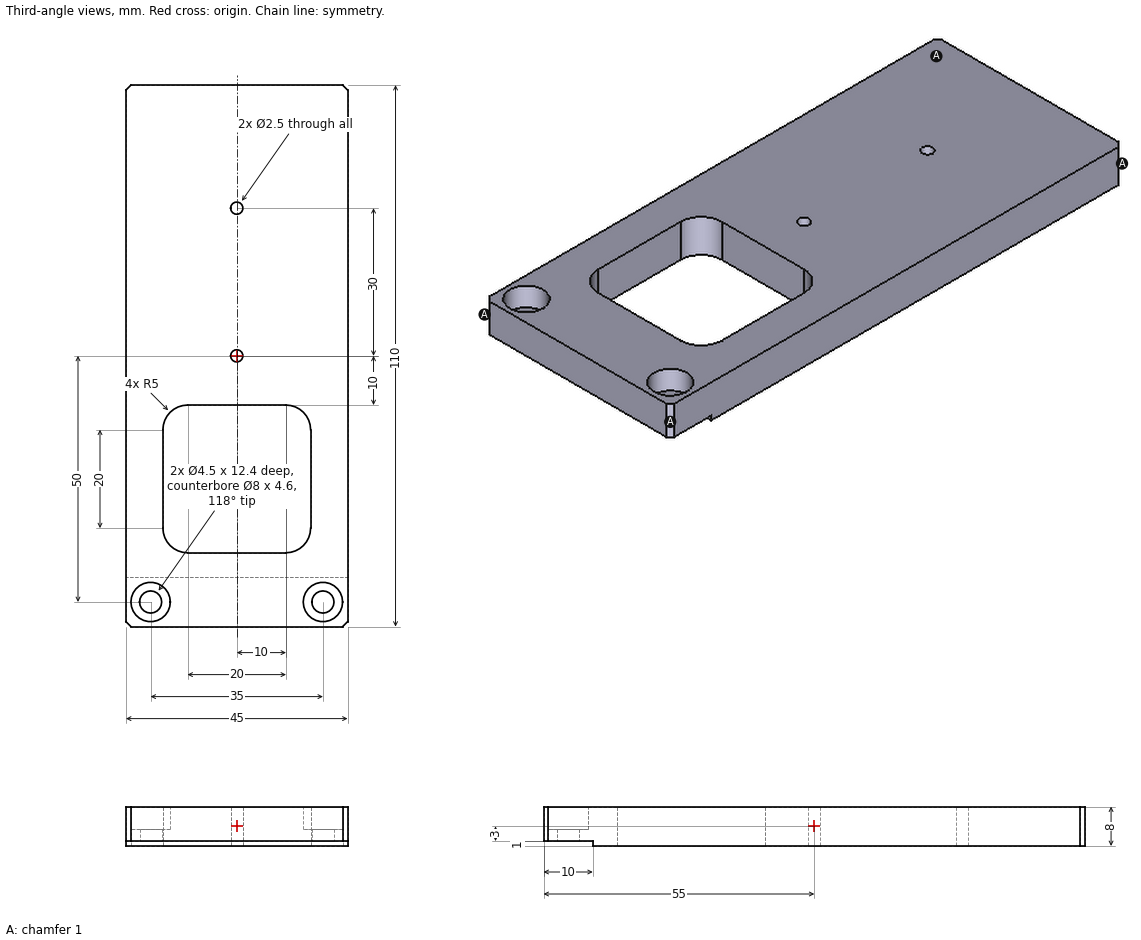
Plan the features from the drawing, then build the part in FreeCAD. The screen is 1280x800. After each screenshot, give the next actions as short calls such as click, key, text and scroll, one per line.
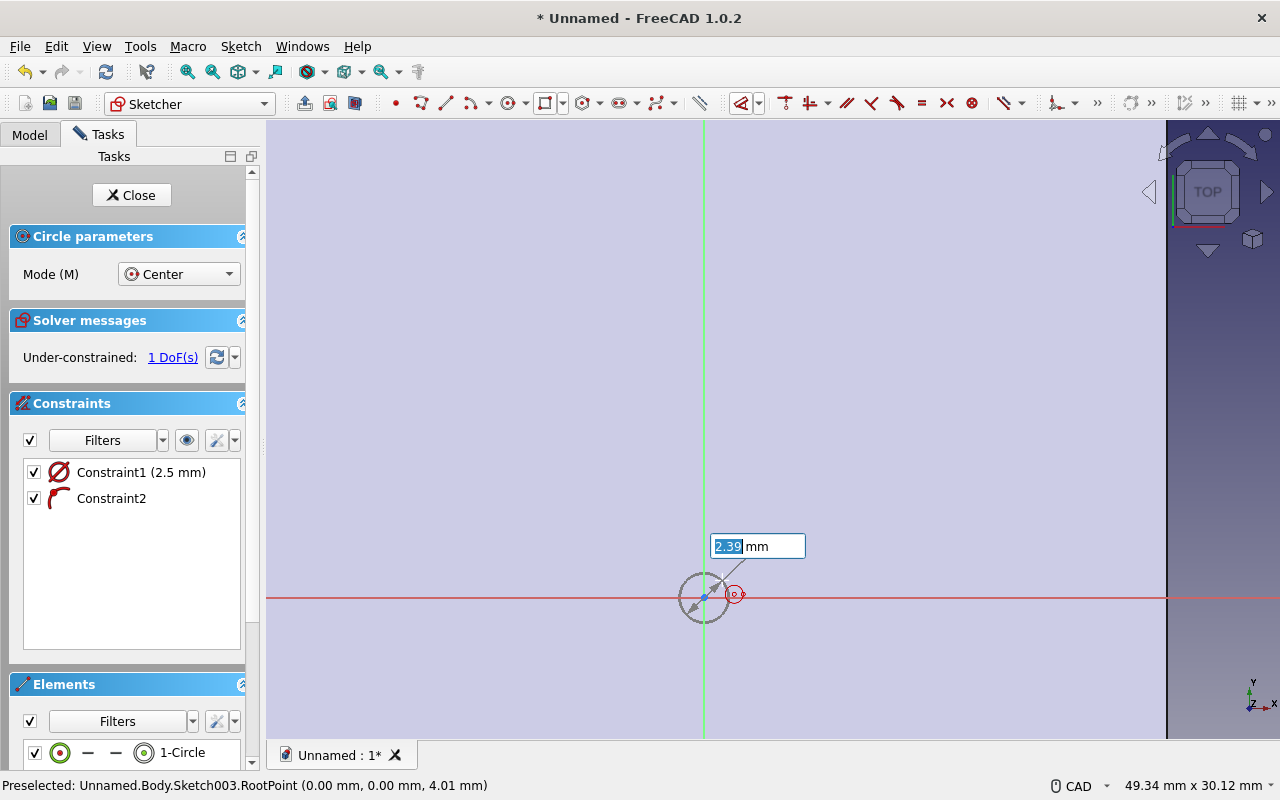
text(2.5)
key(Return)
key(Escape)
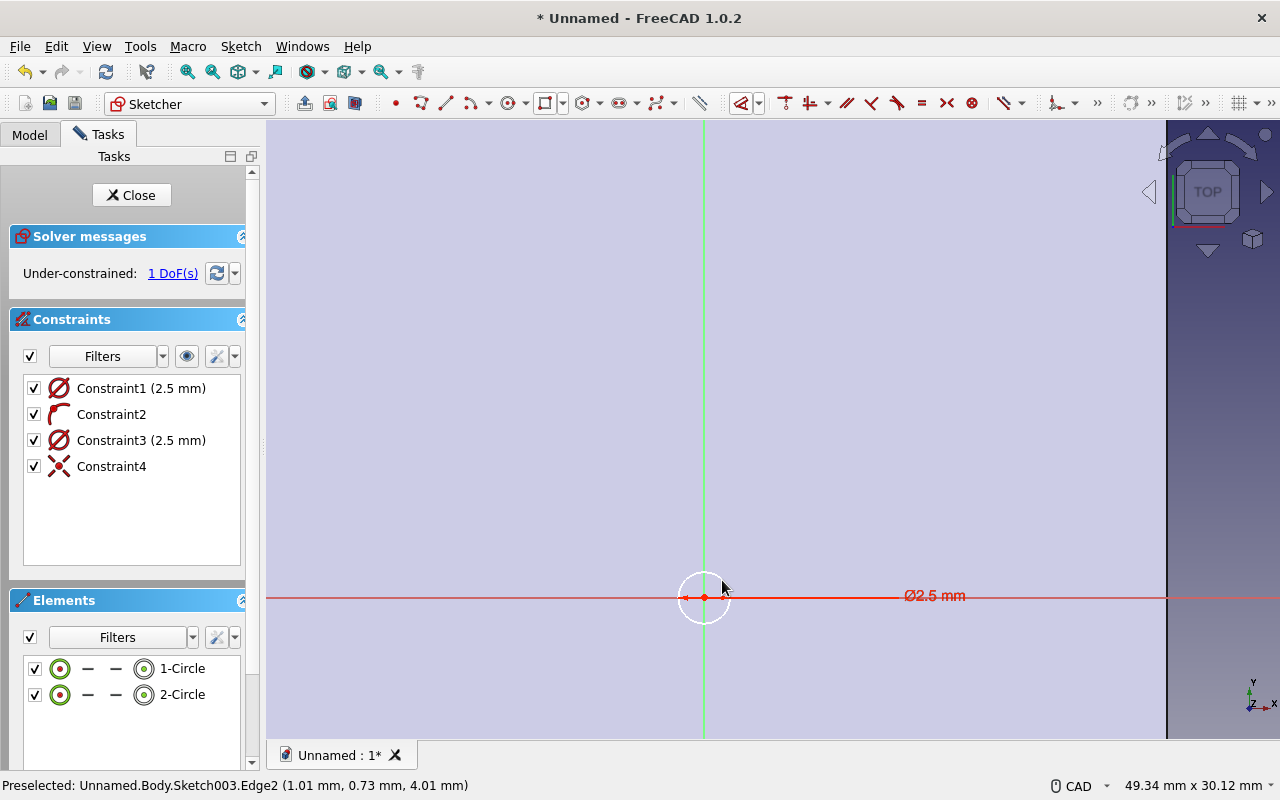
scroll(705, 600, down, 3)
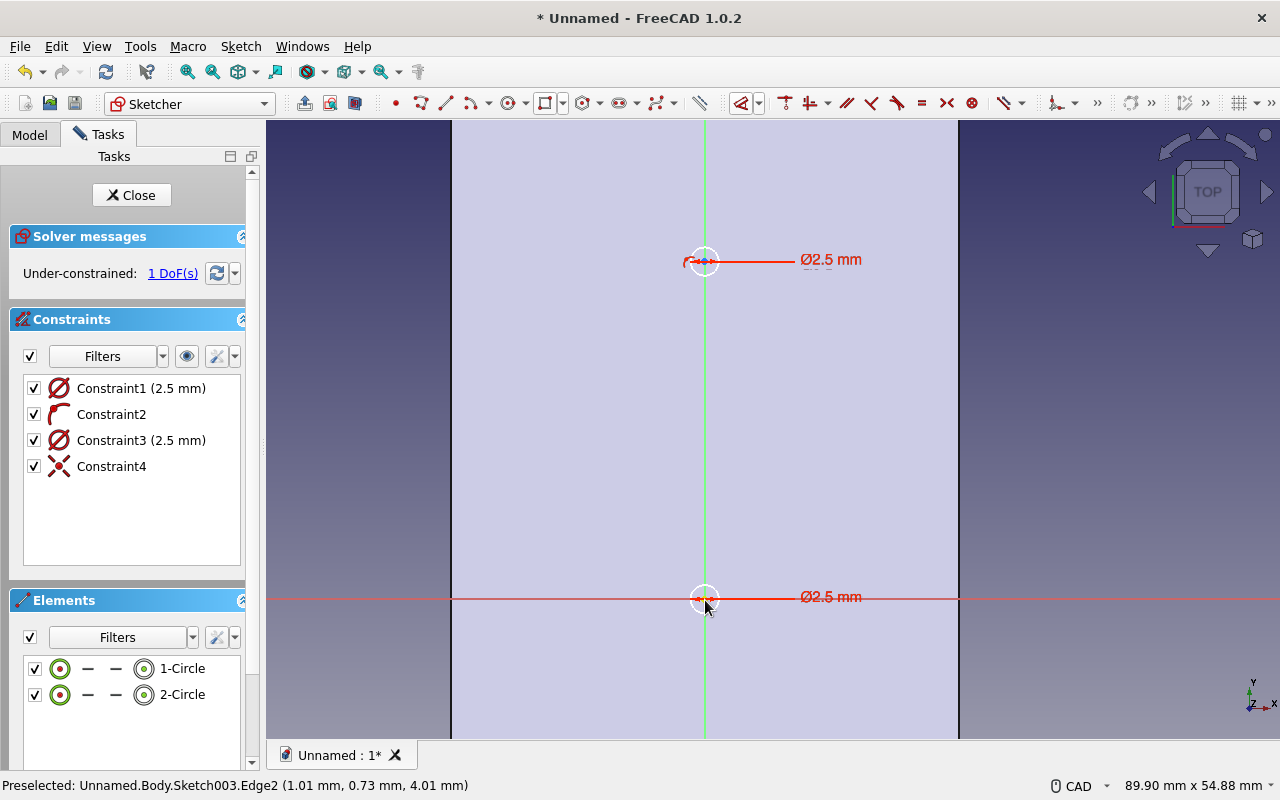
click(705, 262)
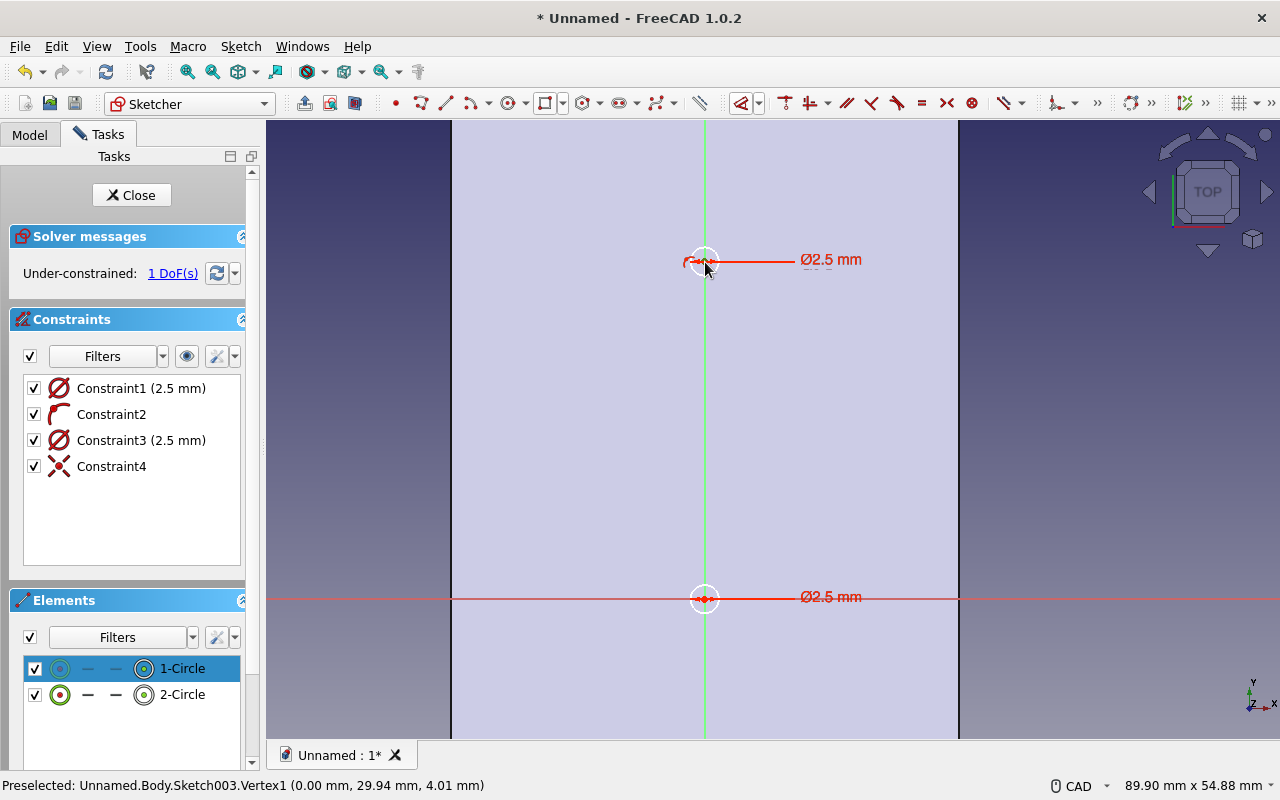
key(i)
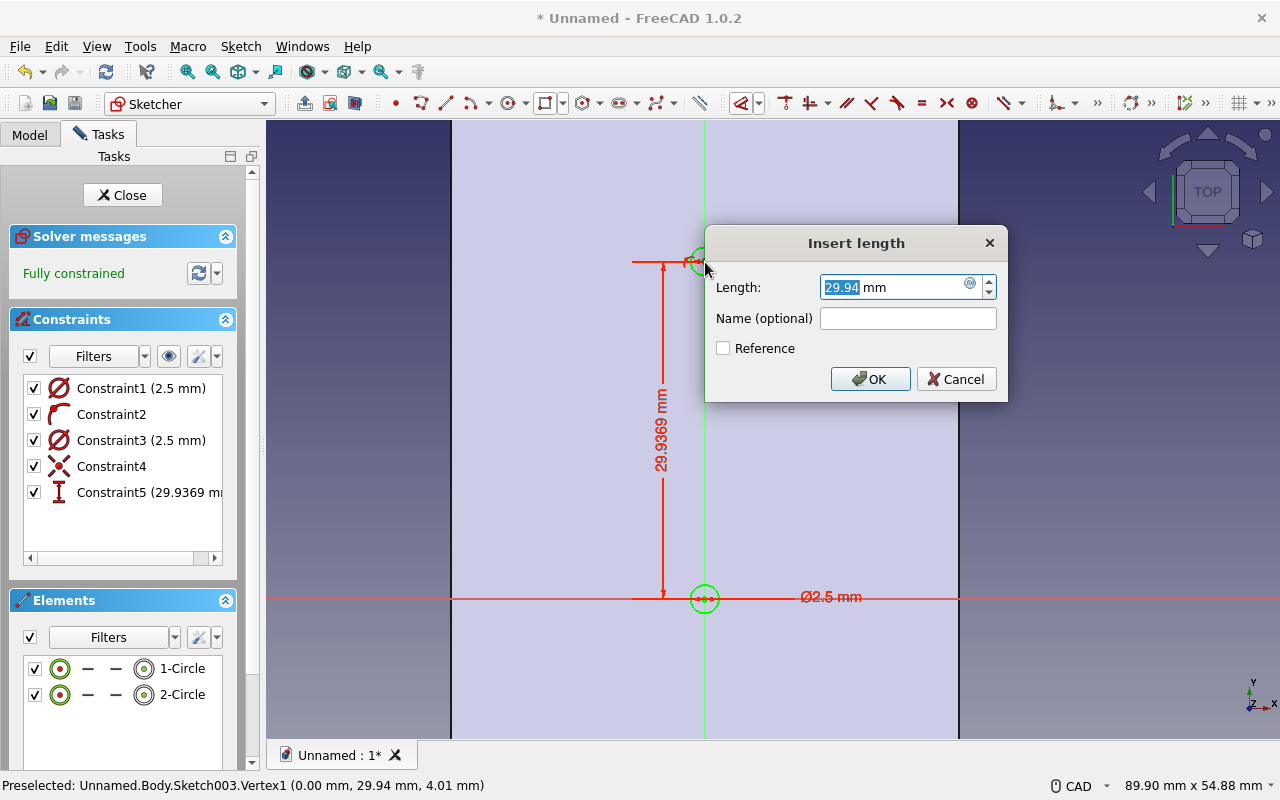
text(30)
key(Return)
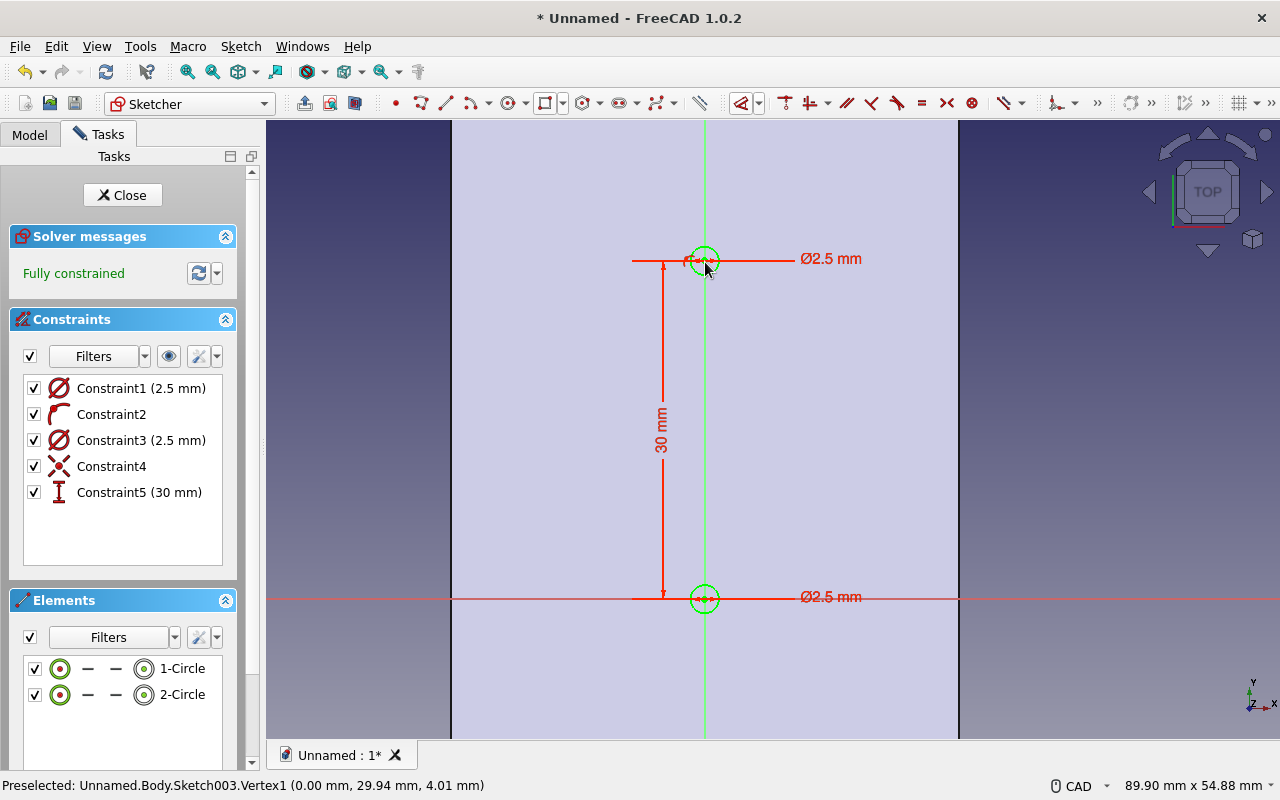
click(123, 195)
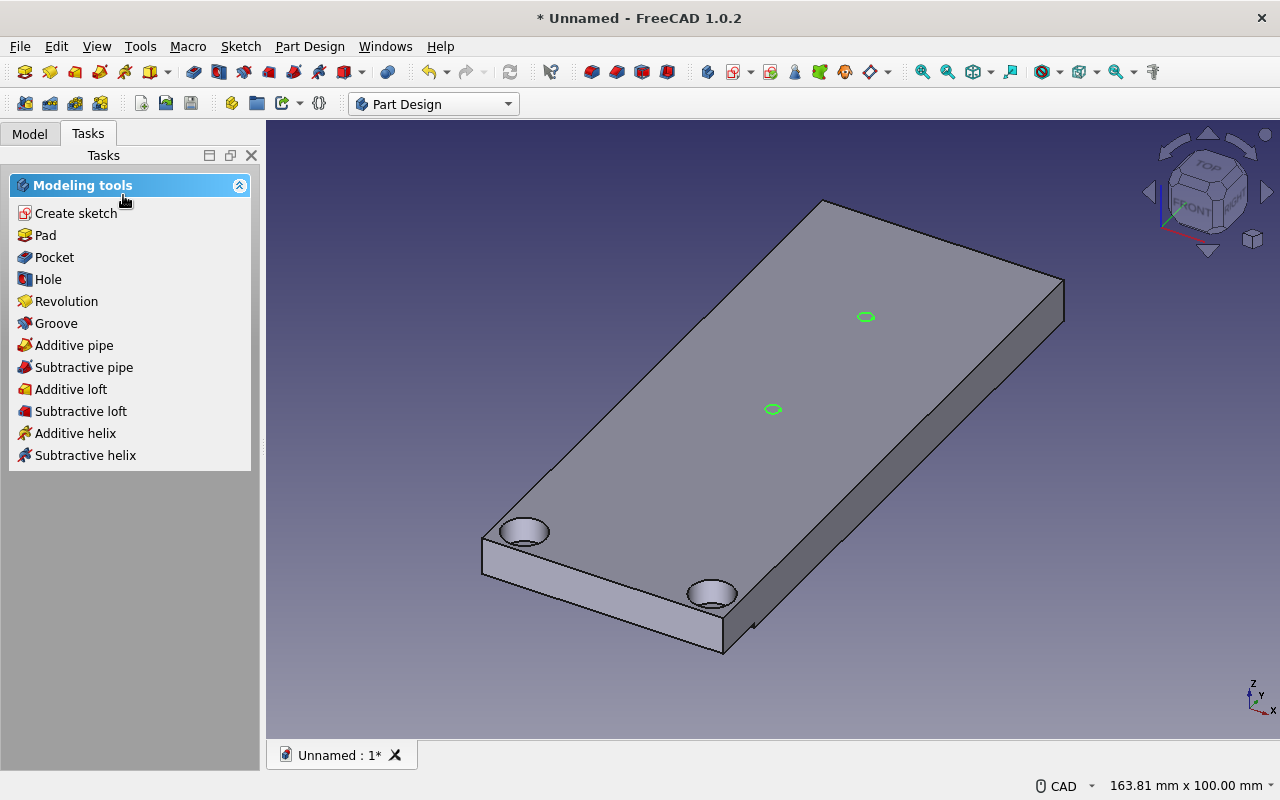
click(219, 72)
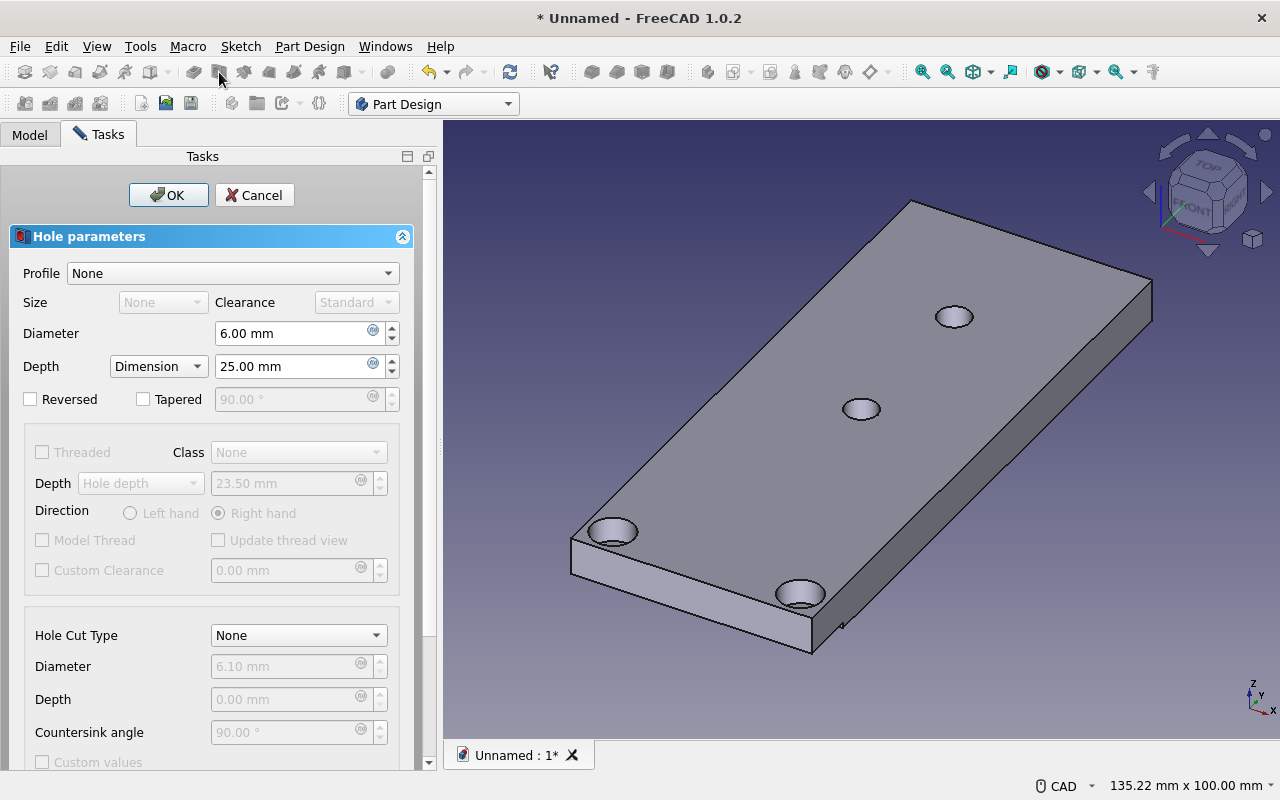
triple_click(300, 334)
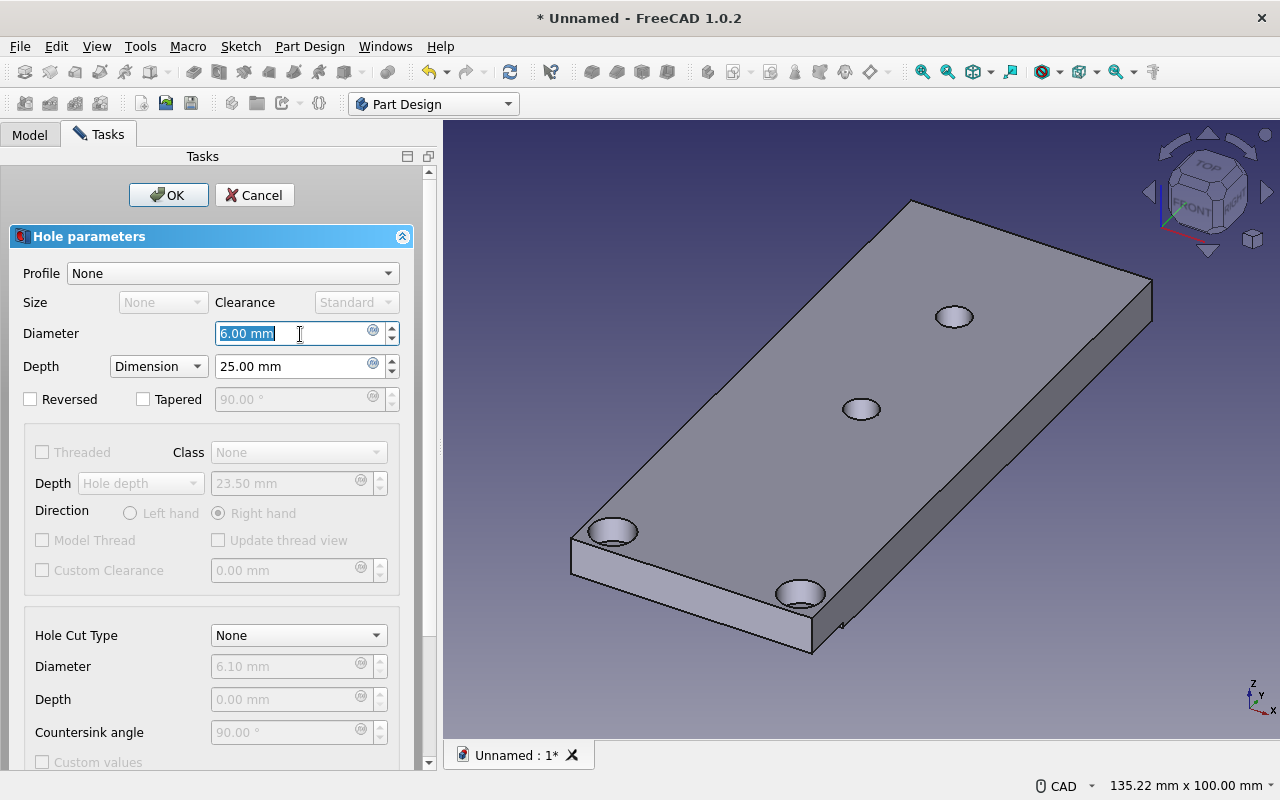
text(2.5)
key(Tab)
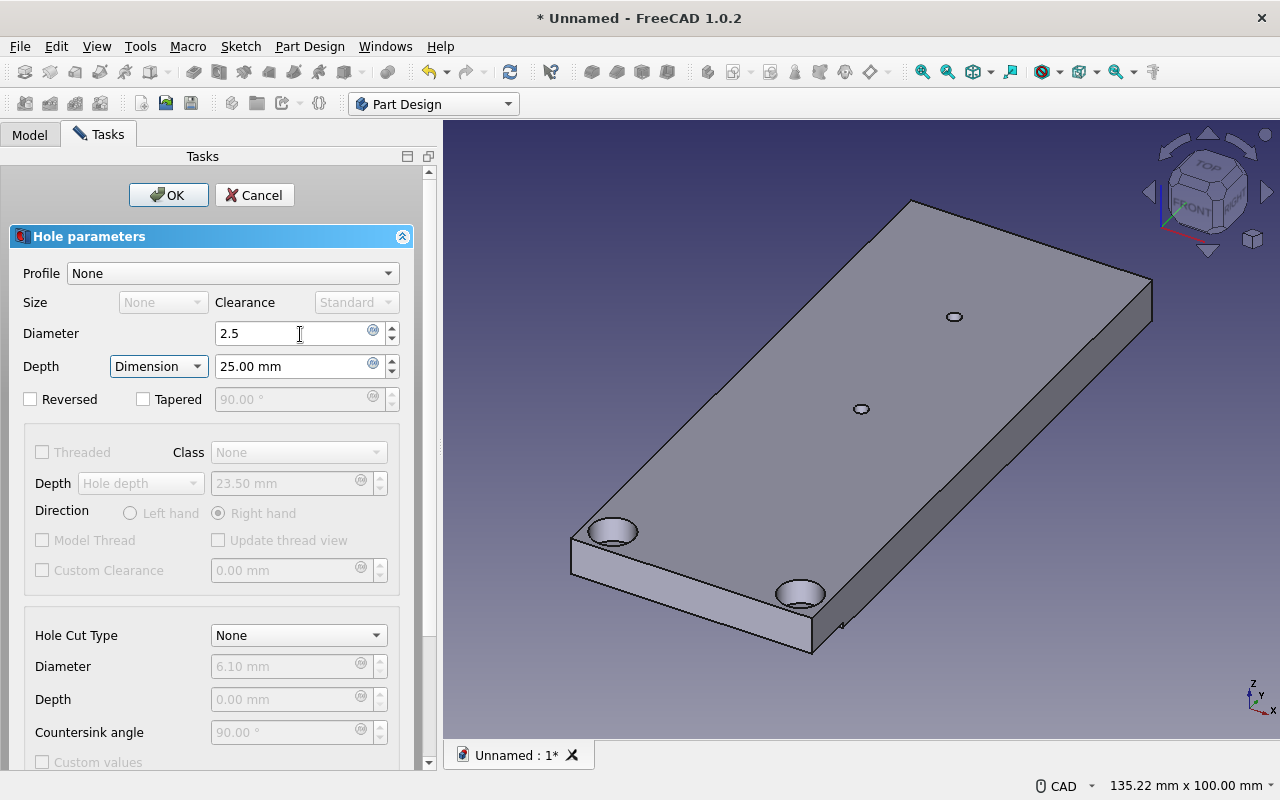
click(160, 366)